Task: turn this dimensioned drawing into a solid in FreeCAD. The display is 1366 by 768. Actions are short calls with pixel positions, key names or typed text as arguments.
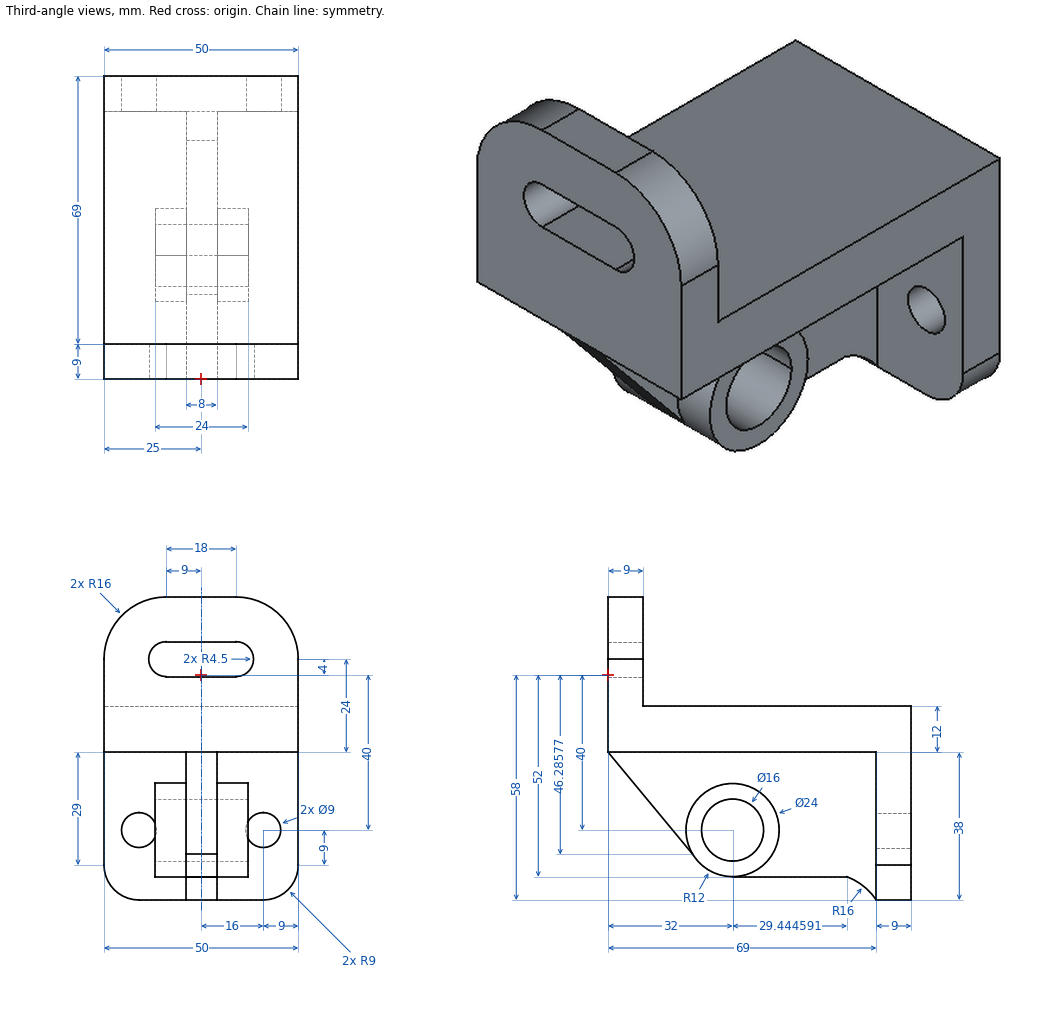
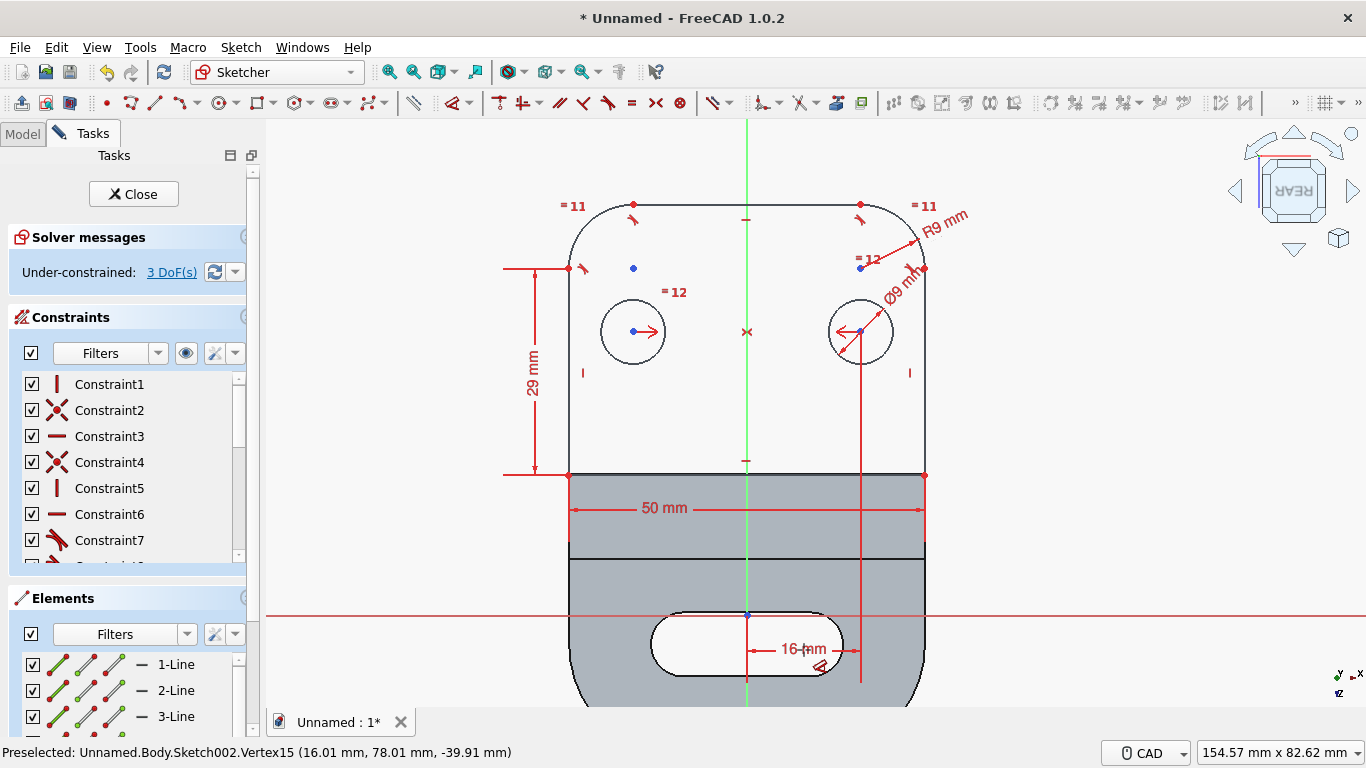
click(861, 332)
click(895, 409)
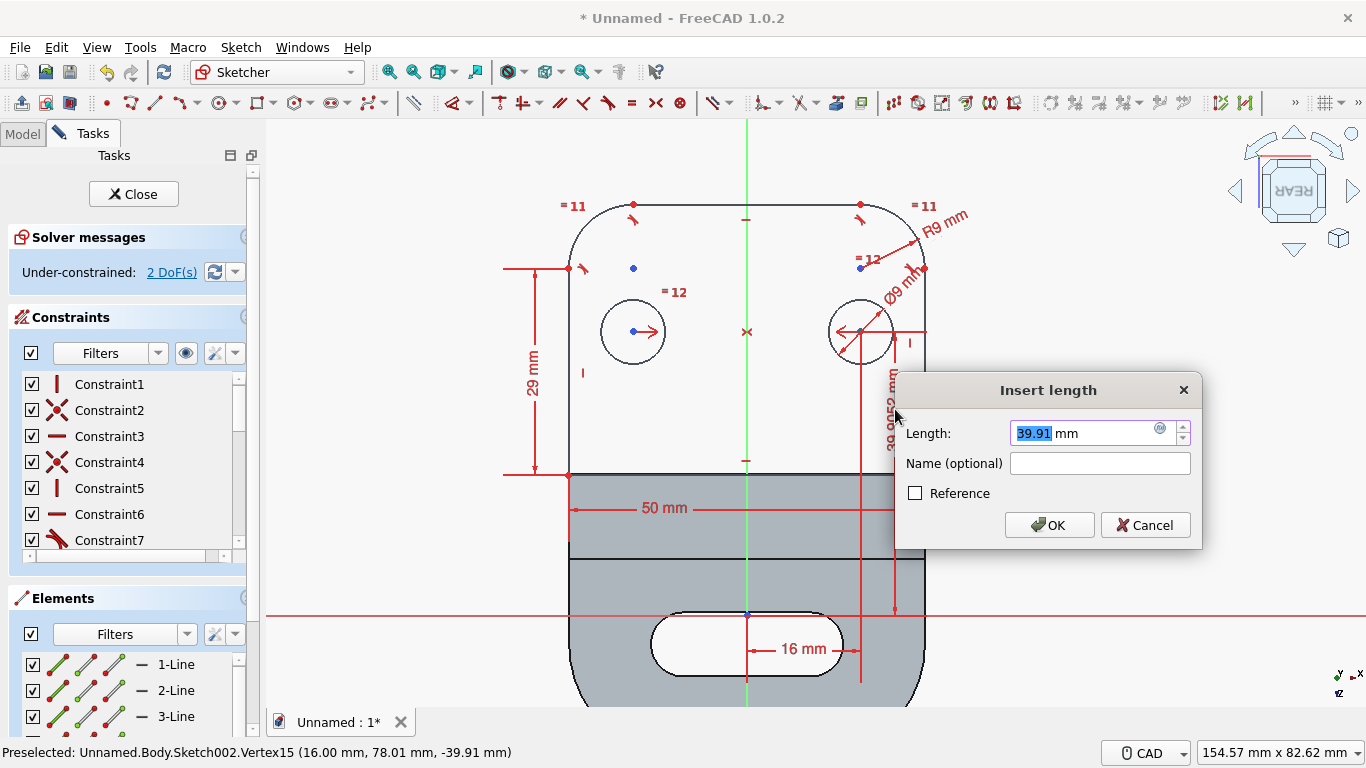
text(40)
key(Return)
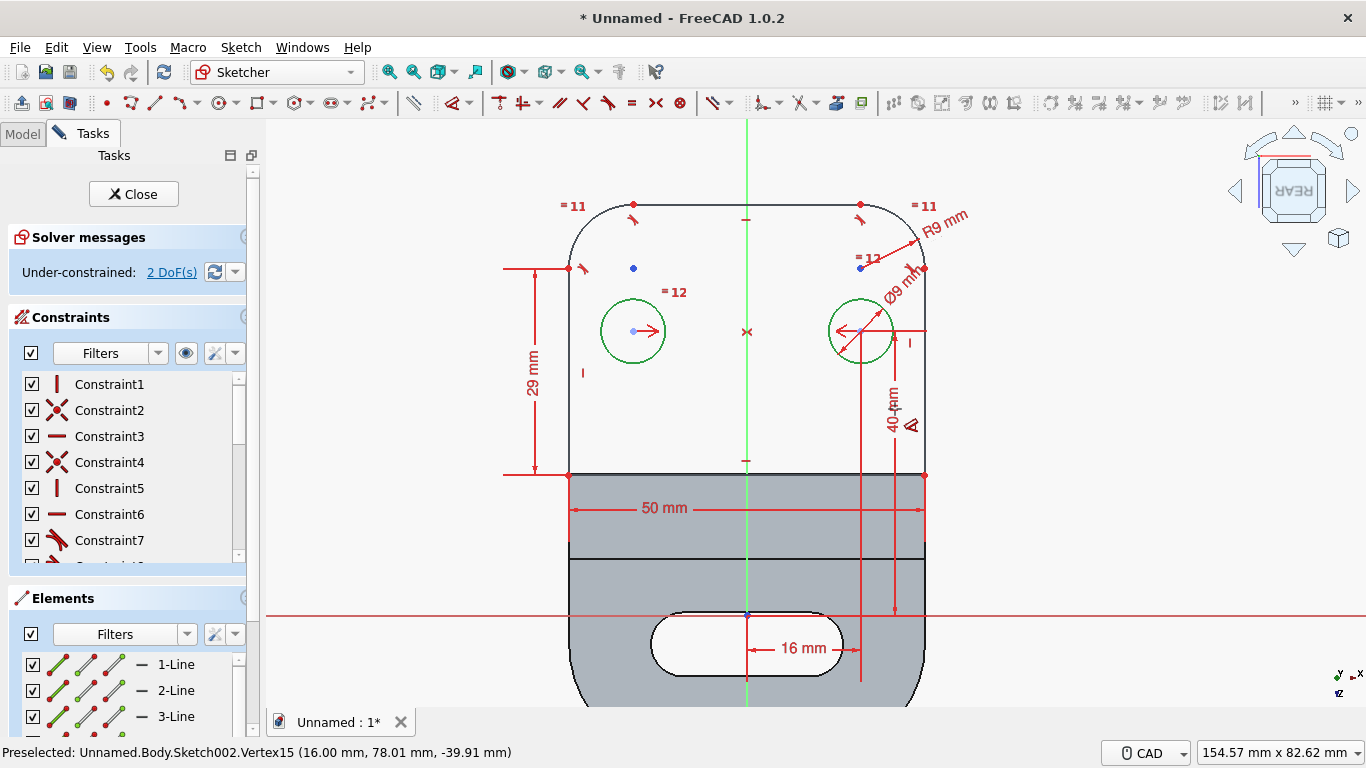
click(925, 269)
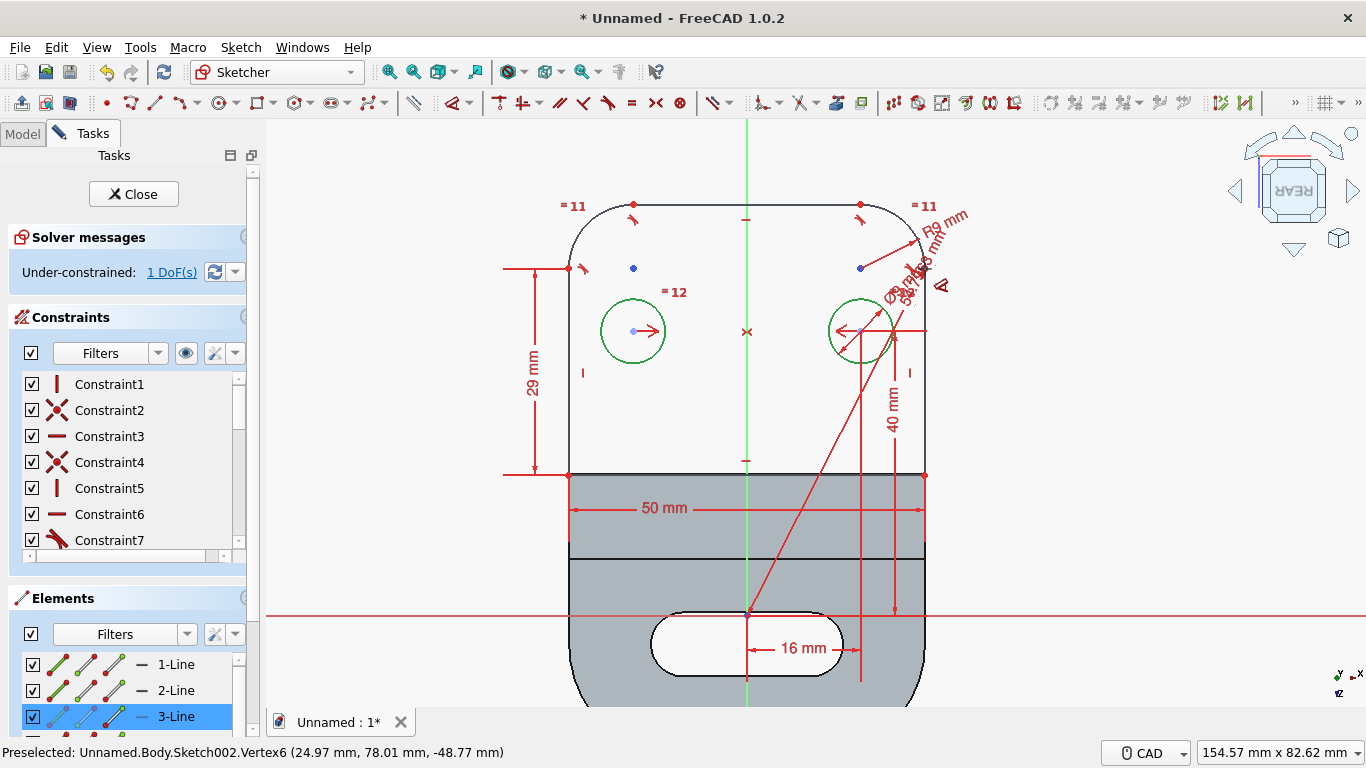
click(861, 331)
click(870, 235)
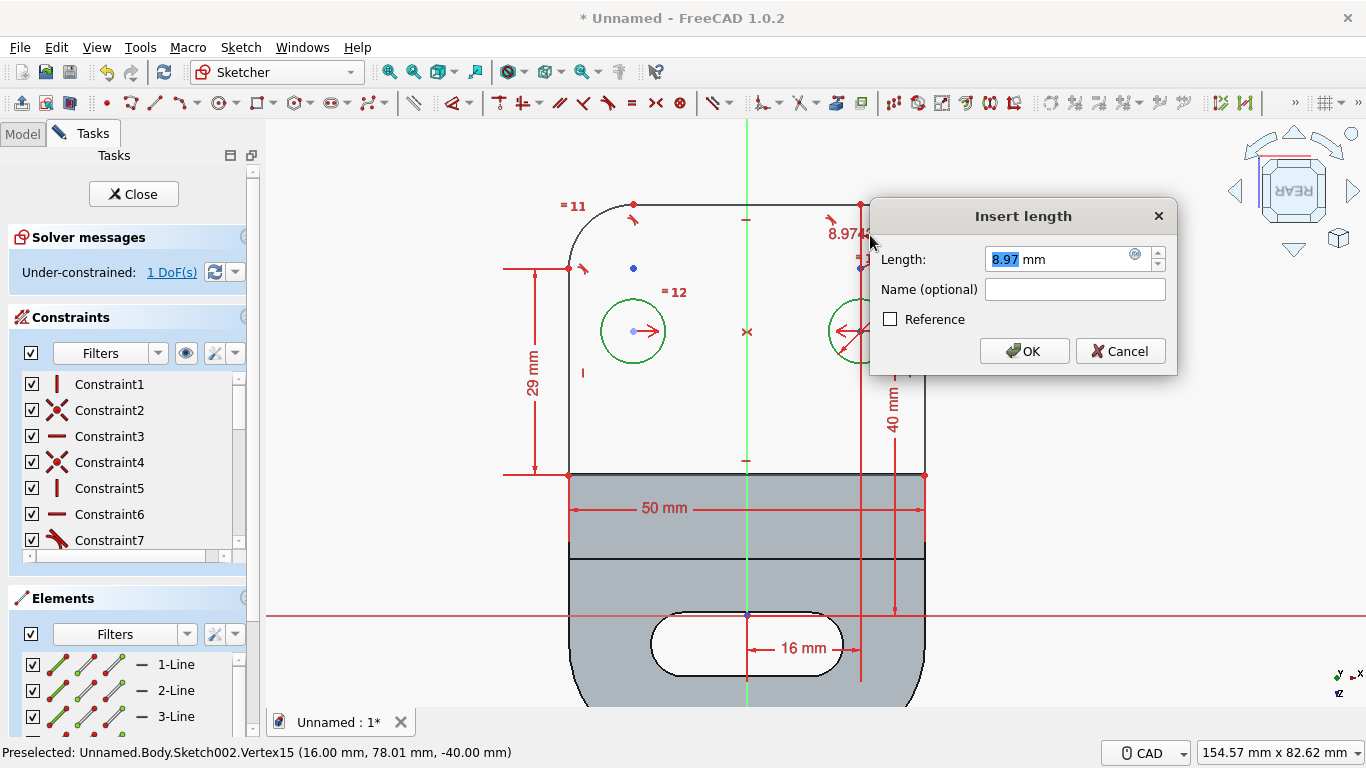
text(9)
key(Return)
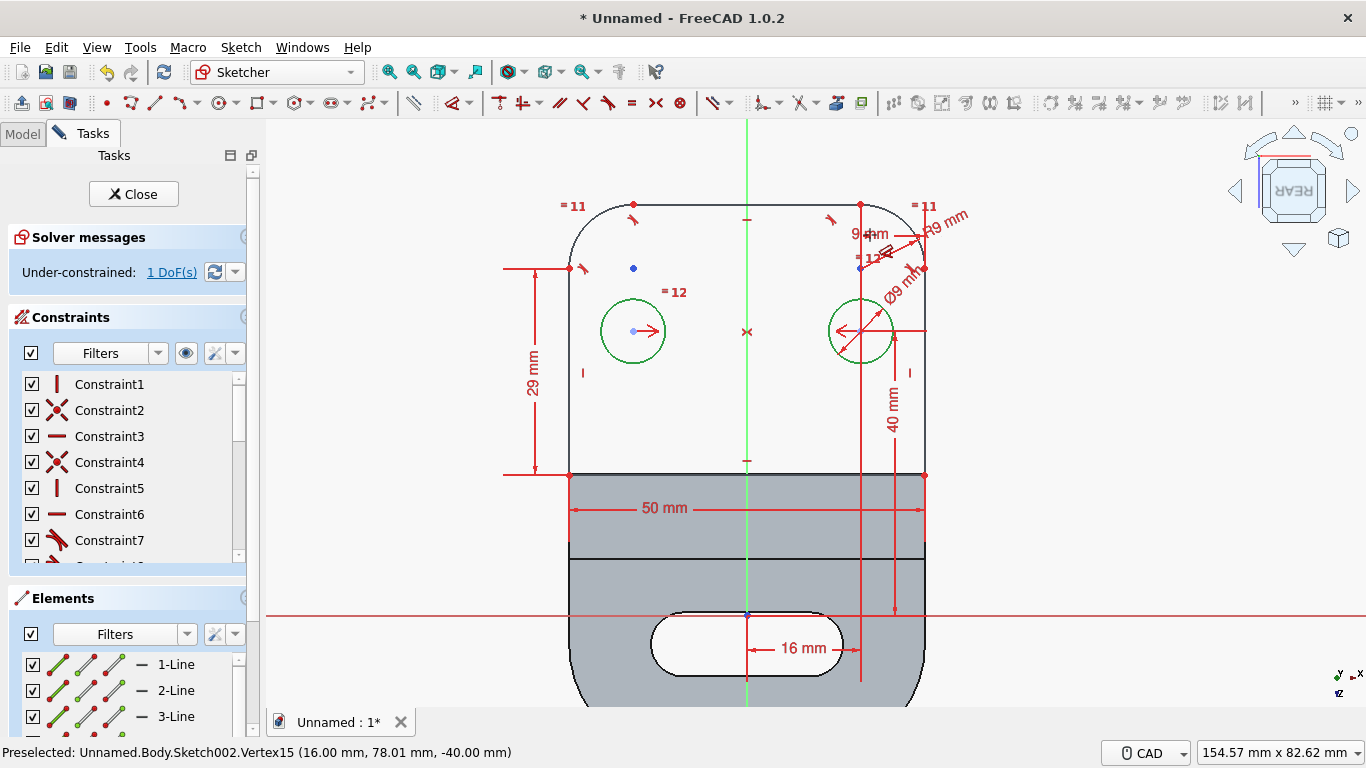
click(925, 269)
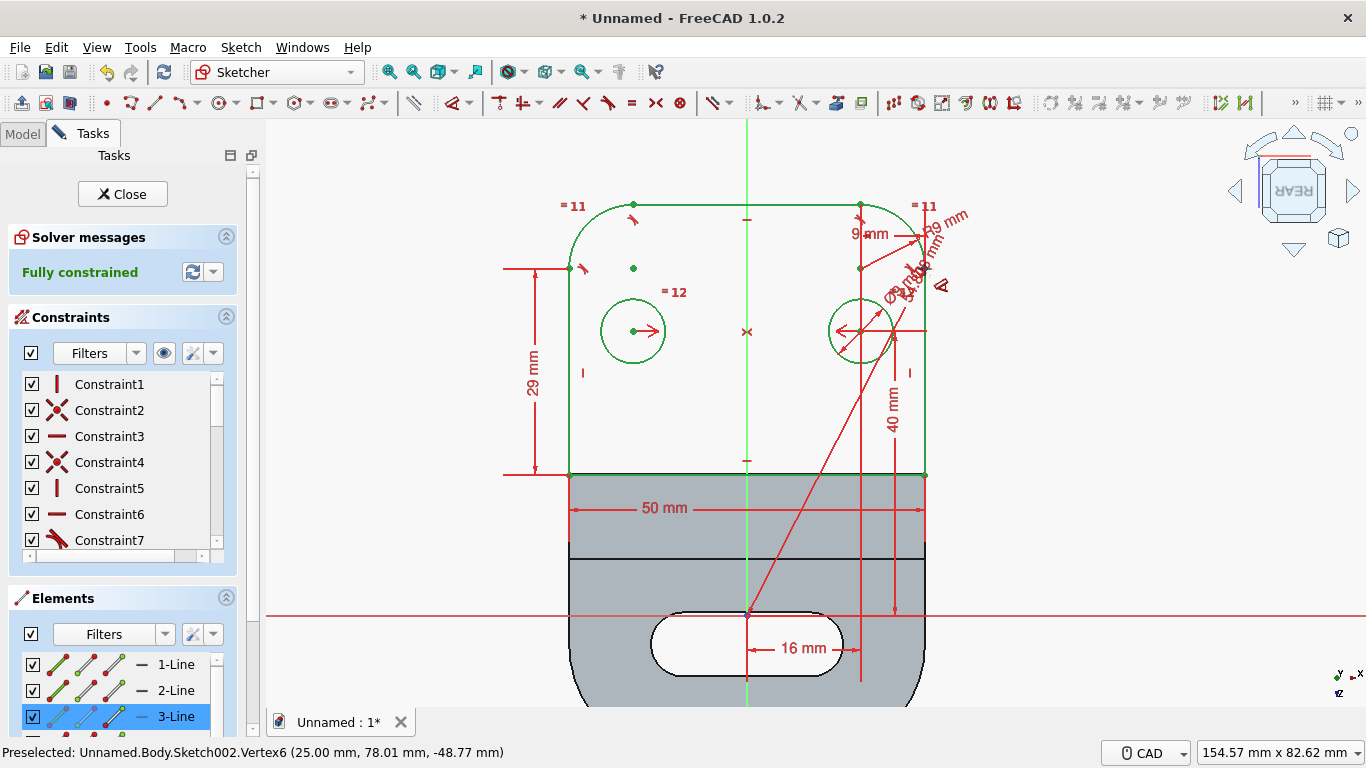
click(861, 331)
click(959, 314)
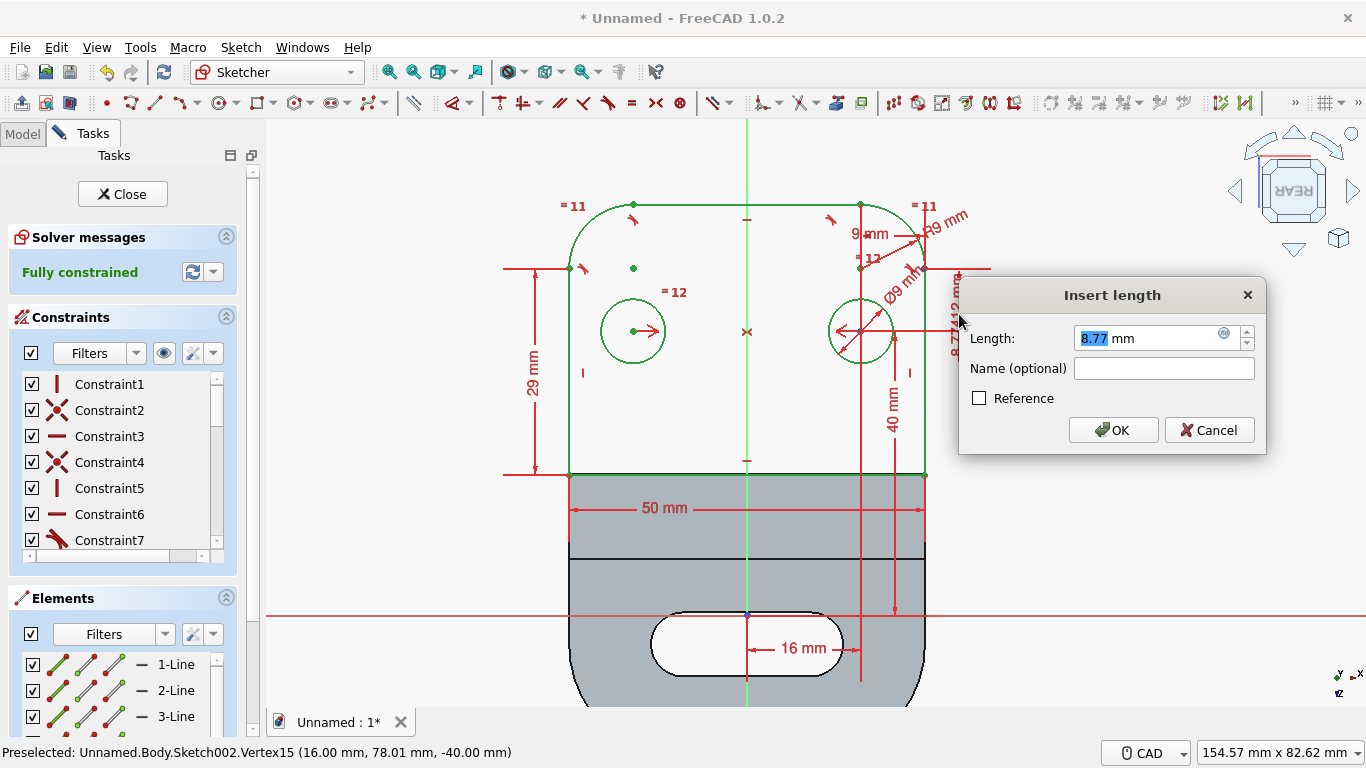
text(9)
key(Return)
key(Escape)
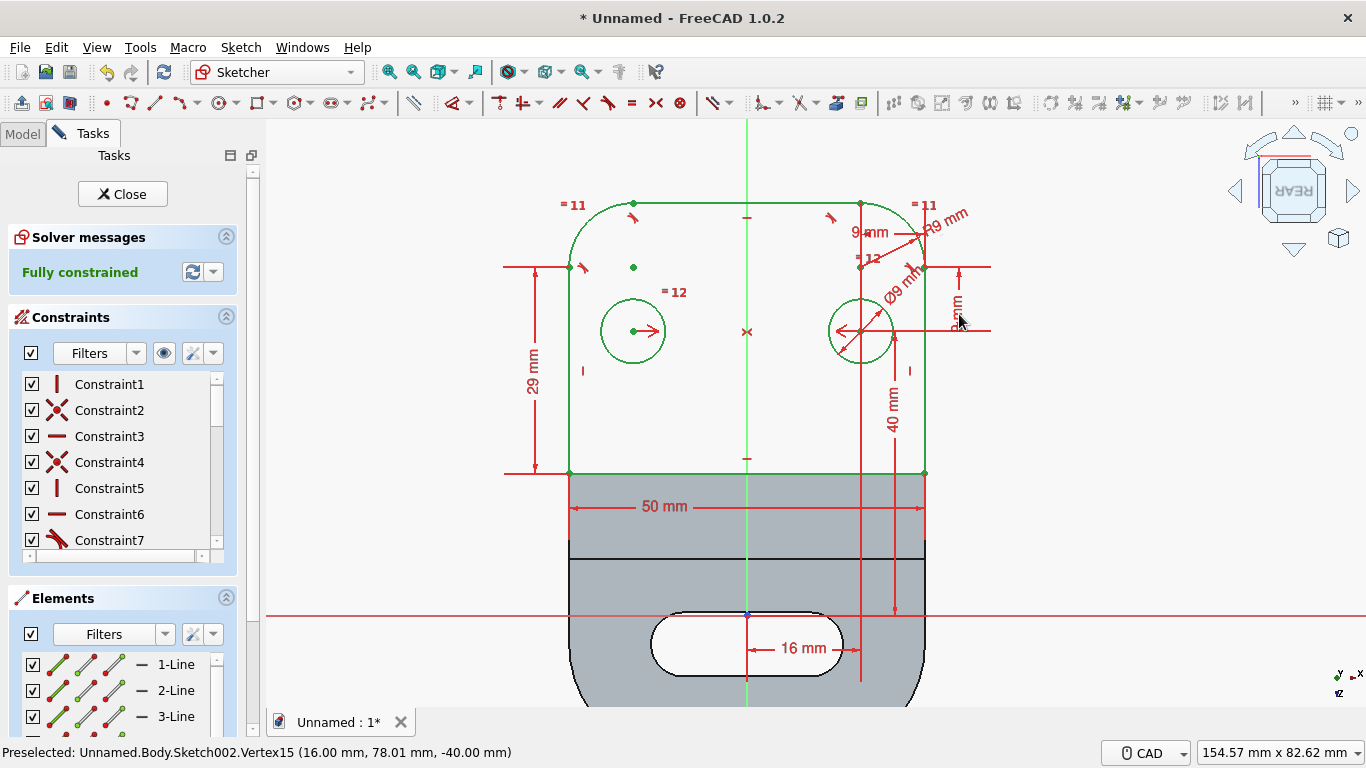
click(123, 194)